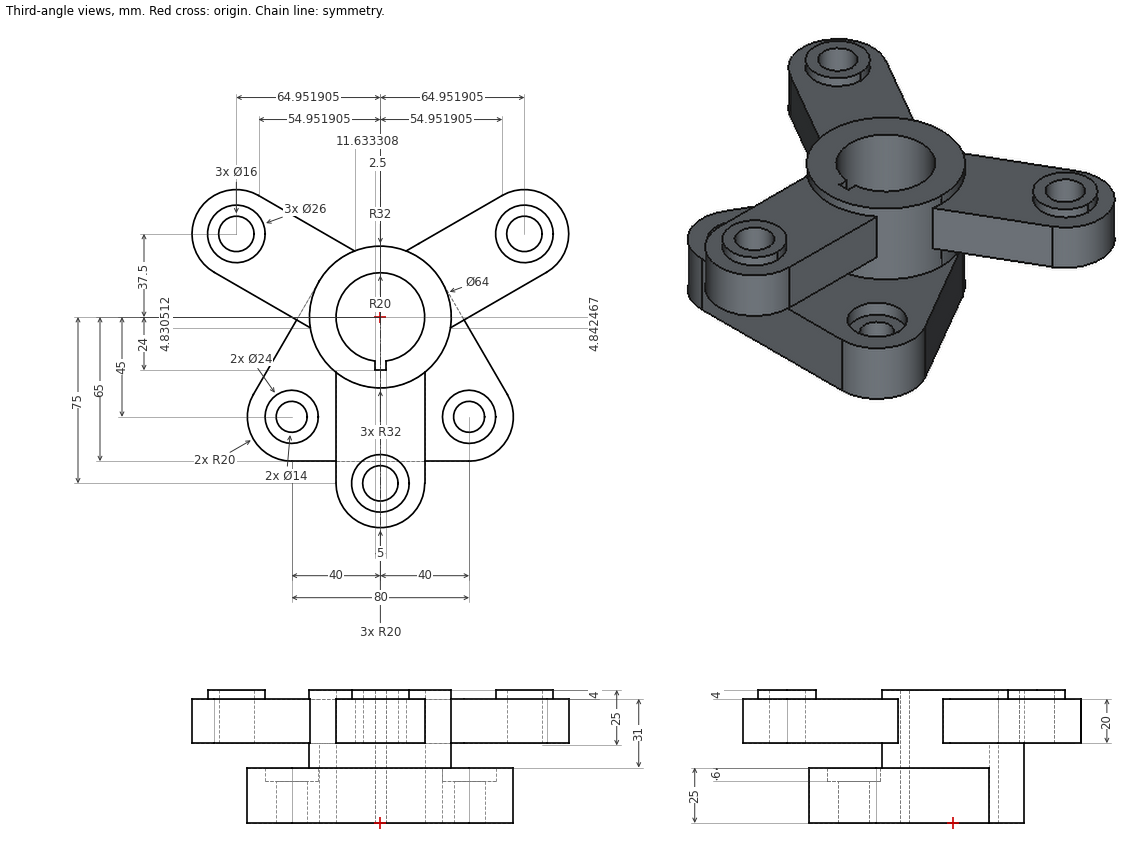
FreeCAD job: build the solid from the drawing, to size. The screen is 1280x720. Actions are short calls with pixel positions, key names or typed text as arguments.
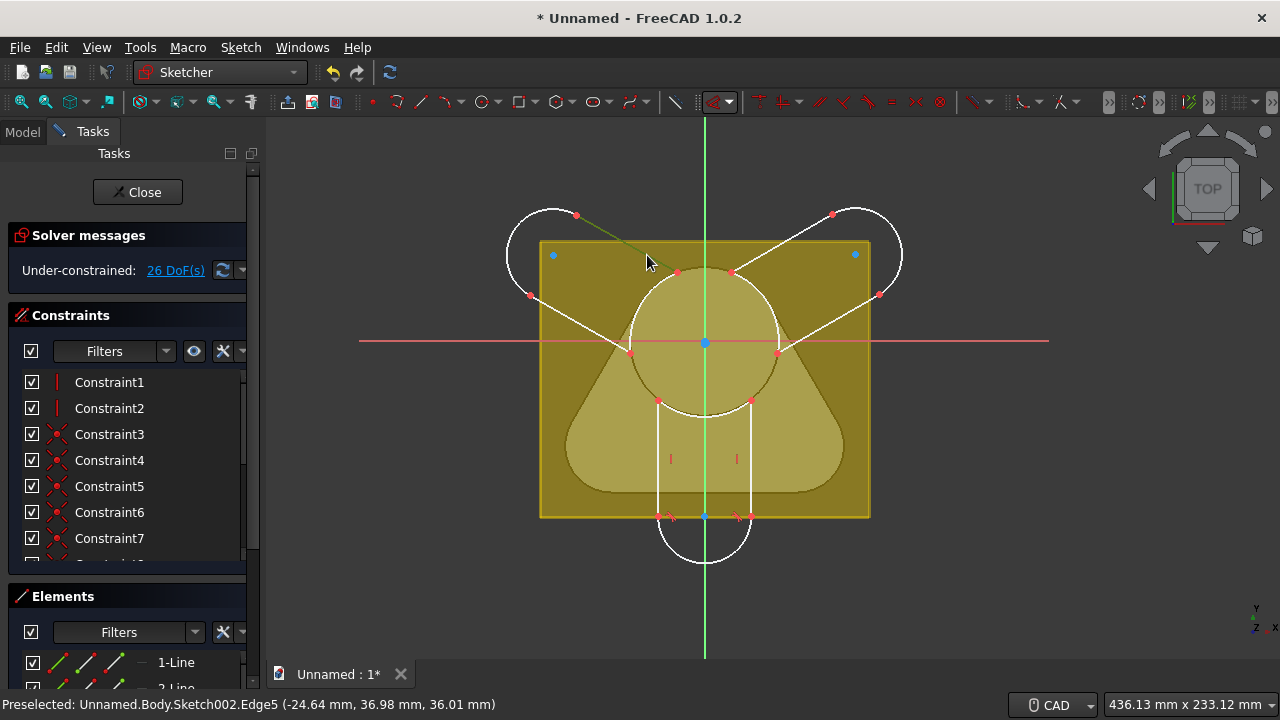
click(534, 213)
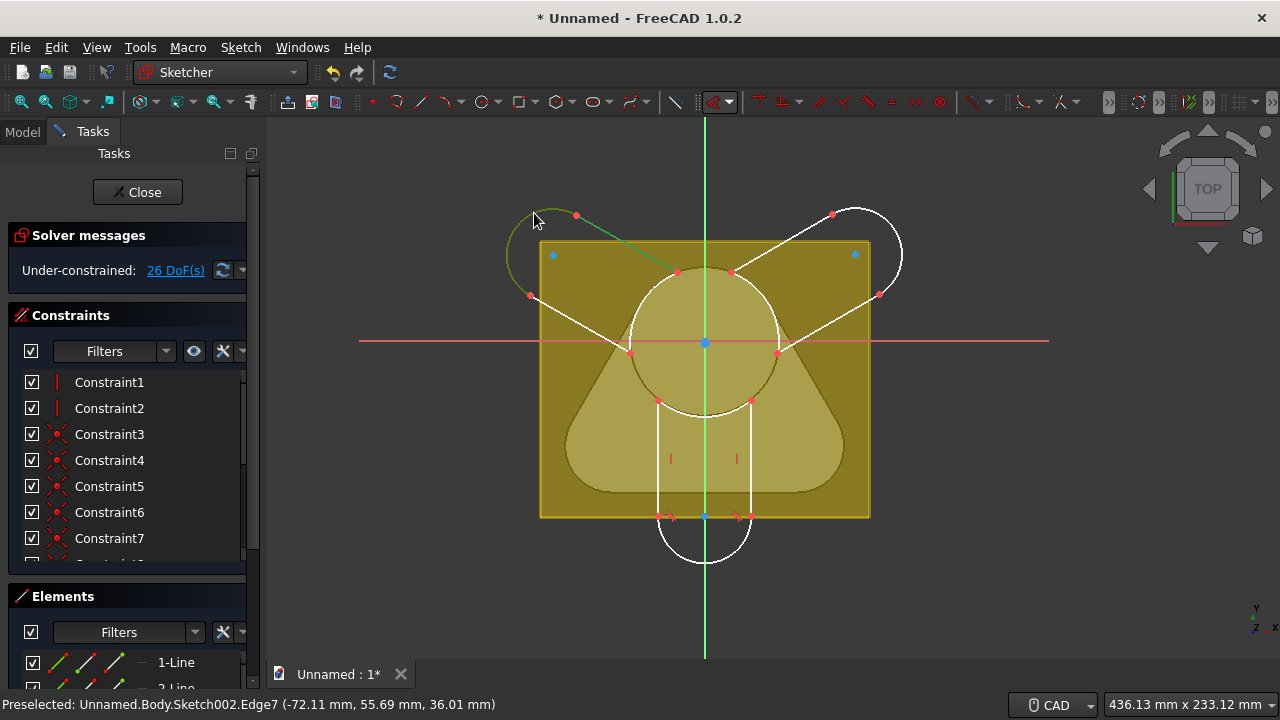
key(t)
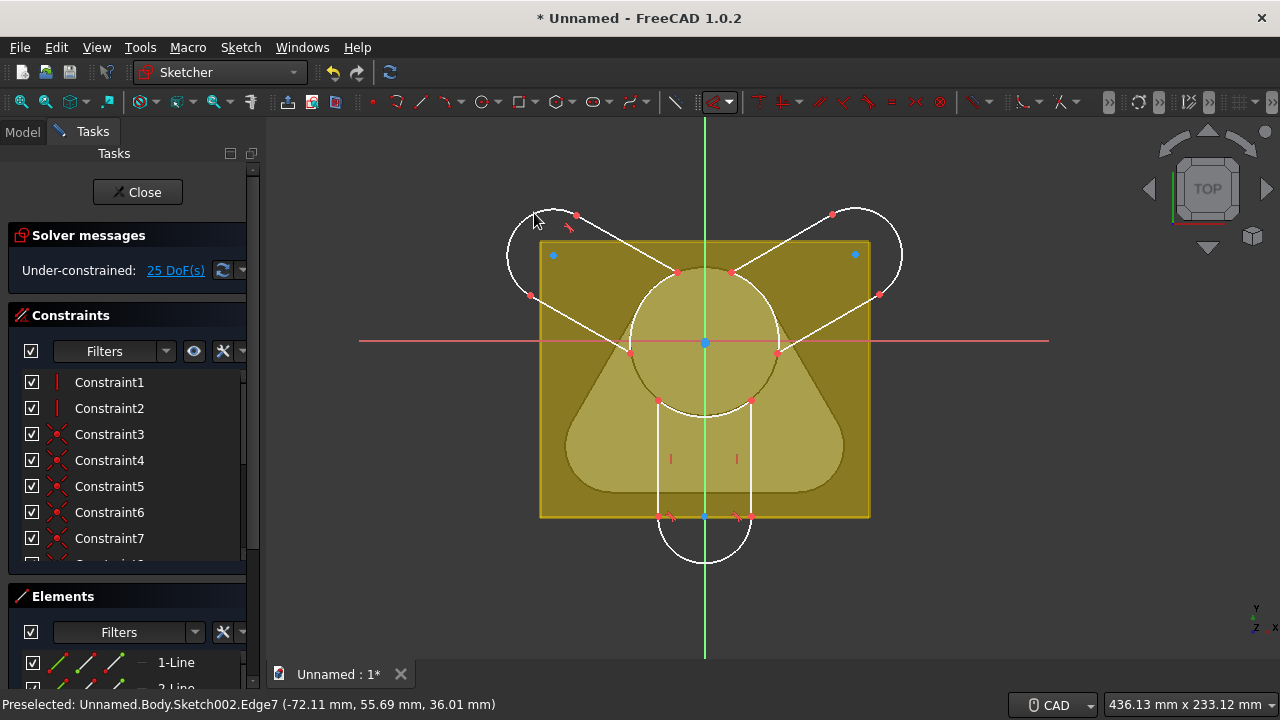
click(560, 313)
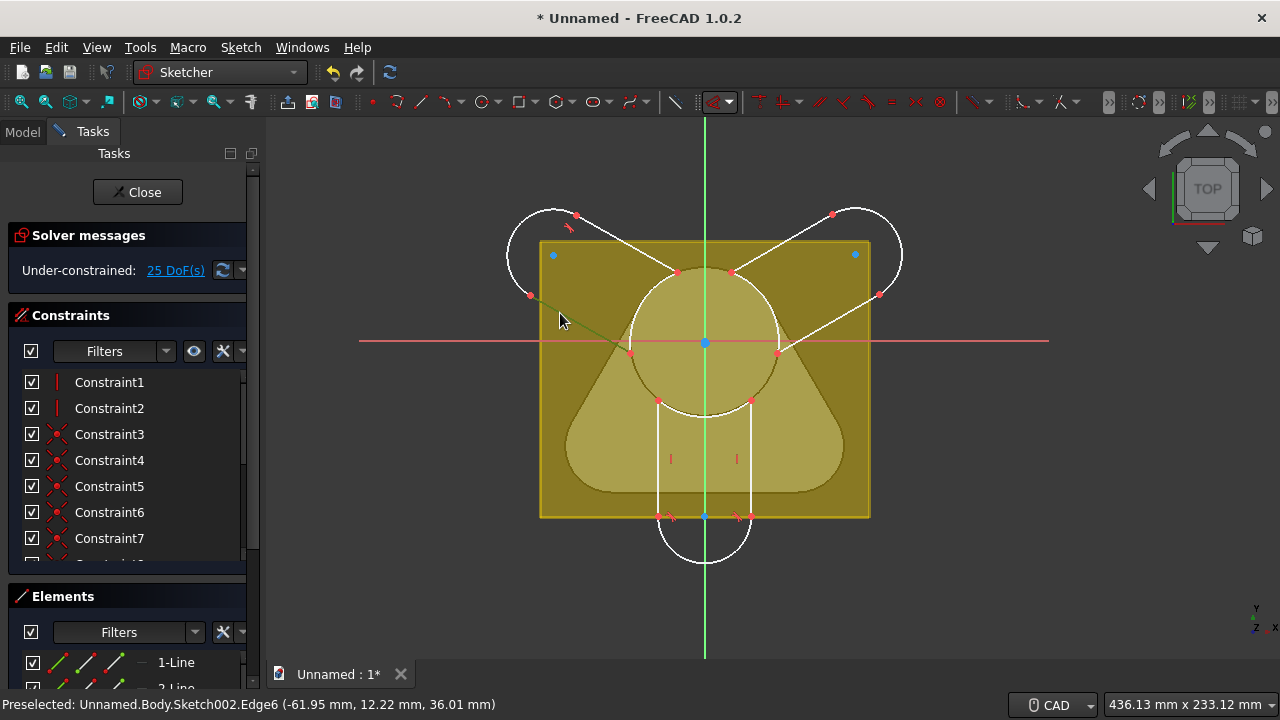
click(535, 214)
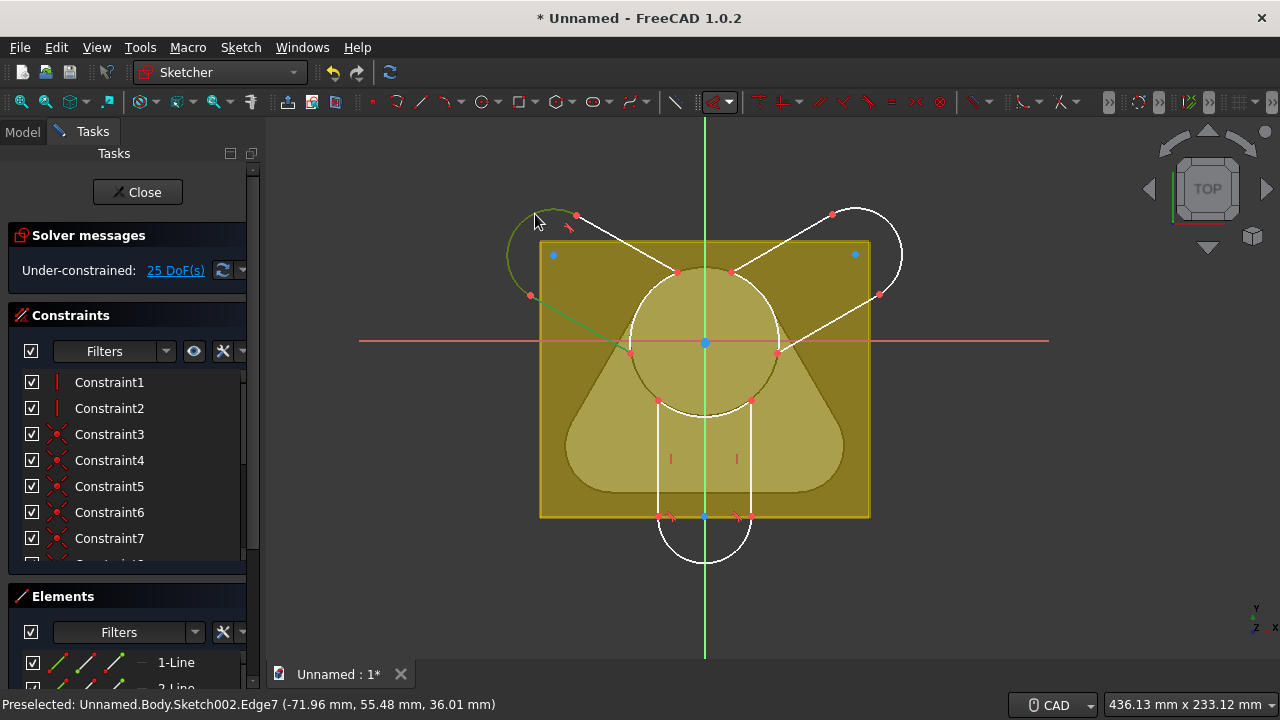
key(t)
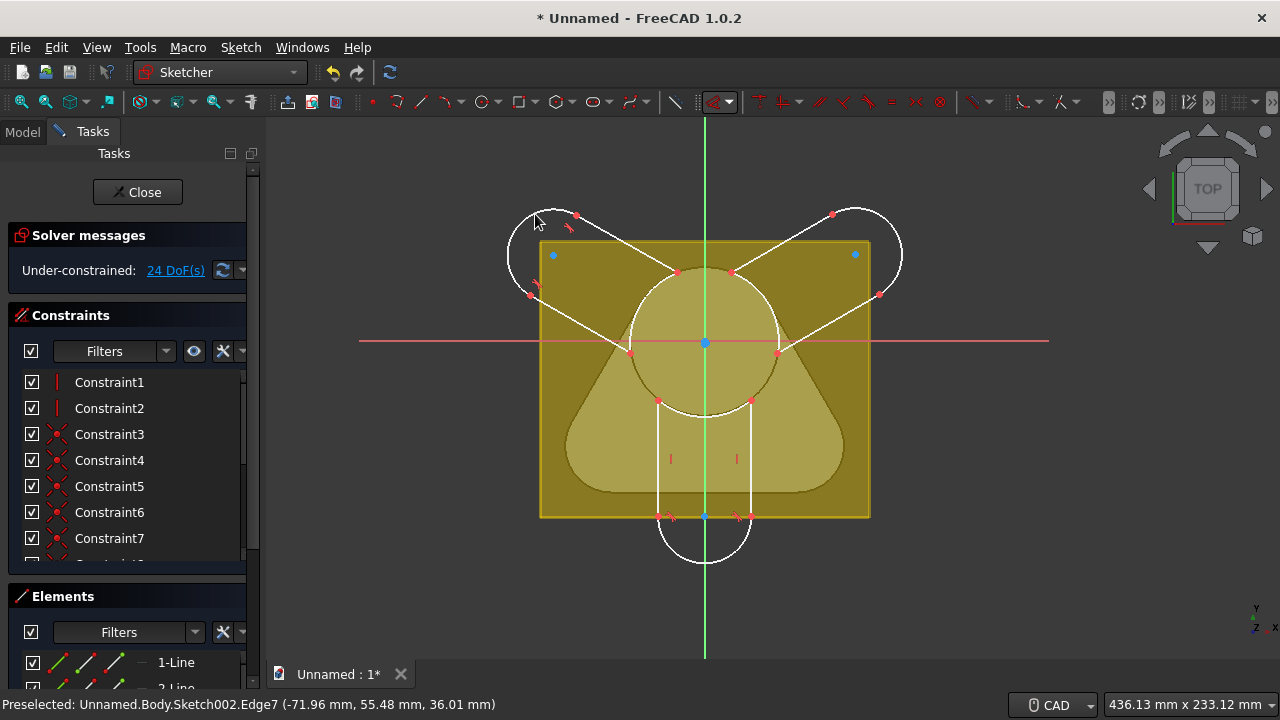
click(802, 232)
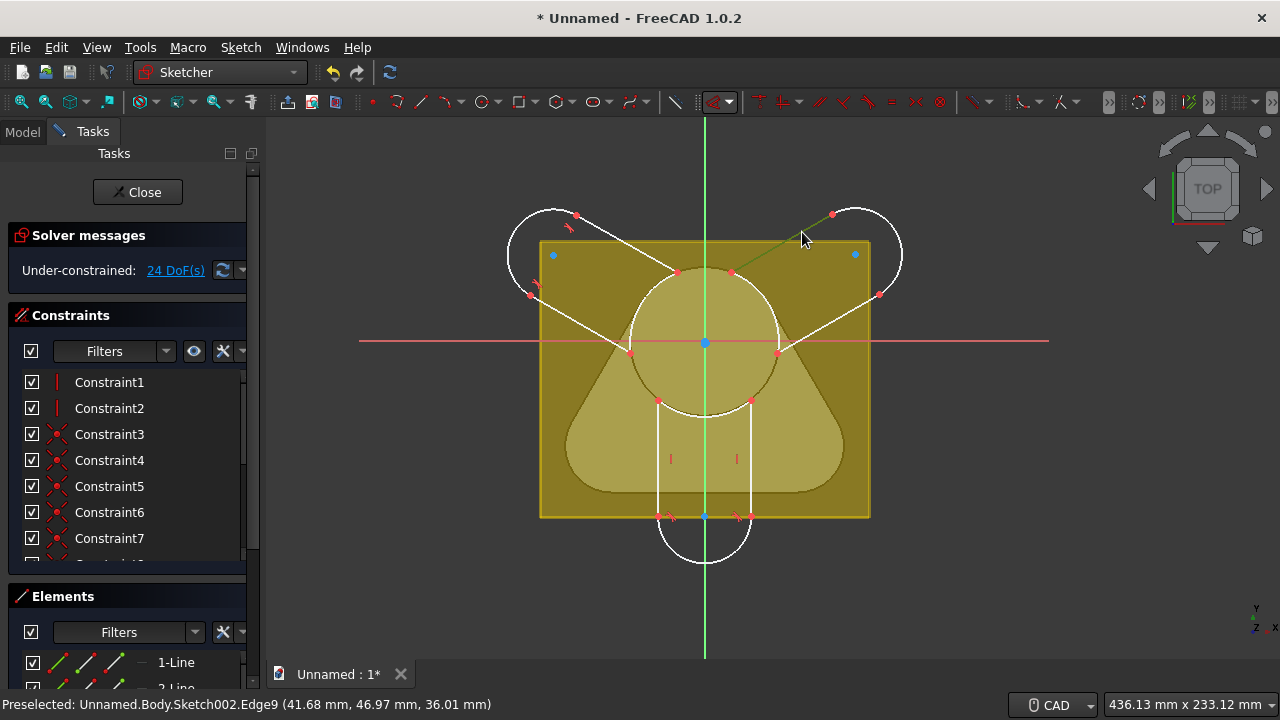
click(902, 259)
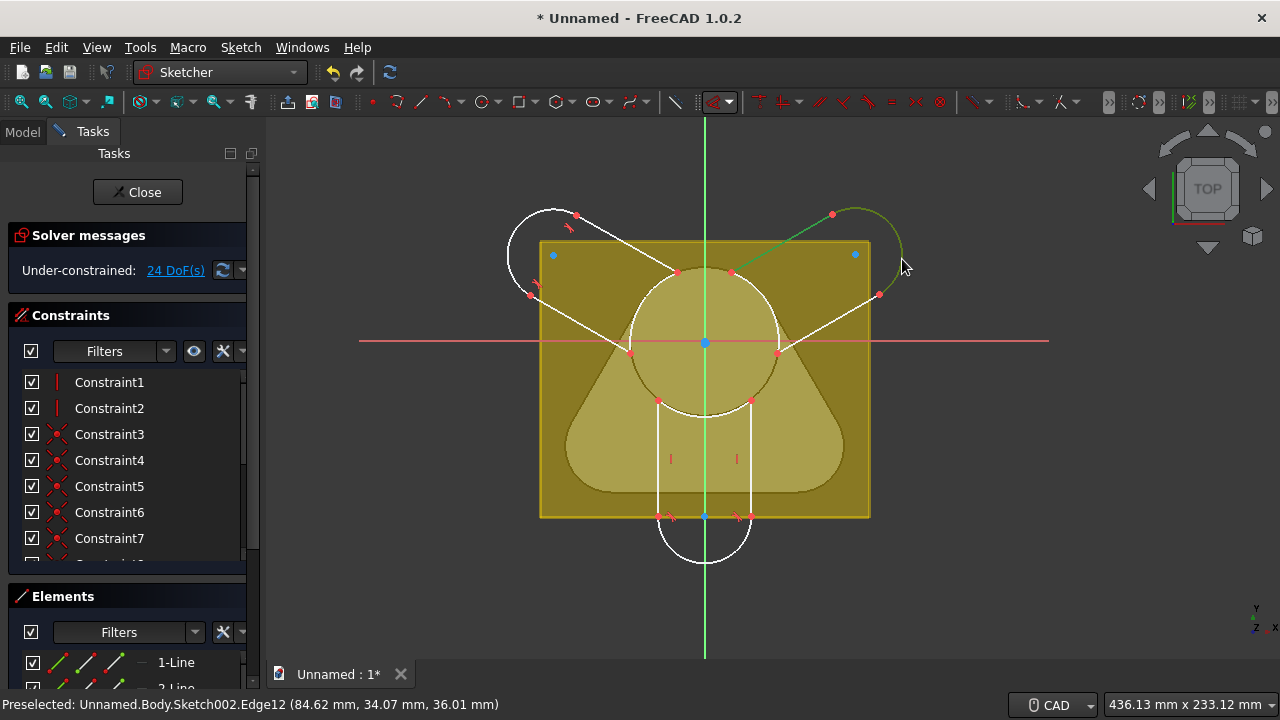
key(t)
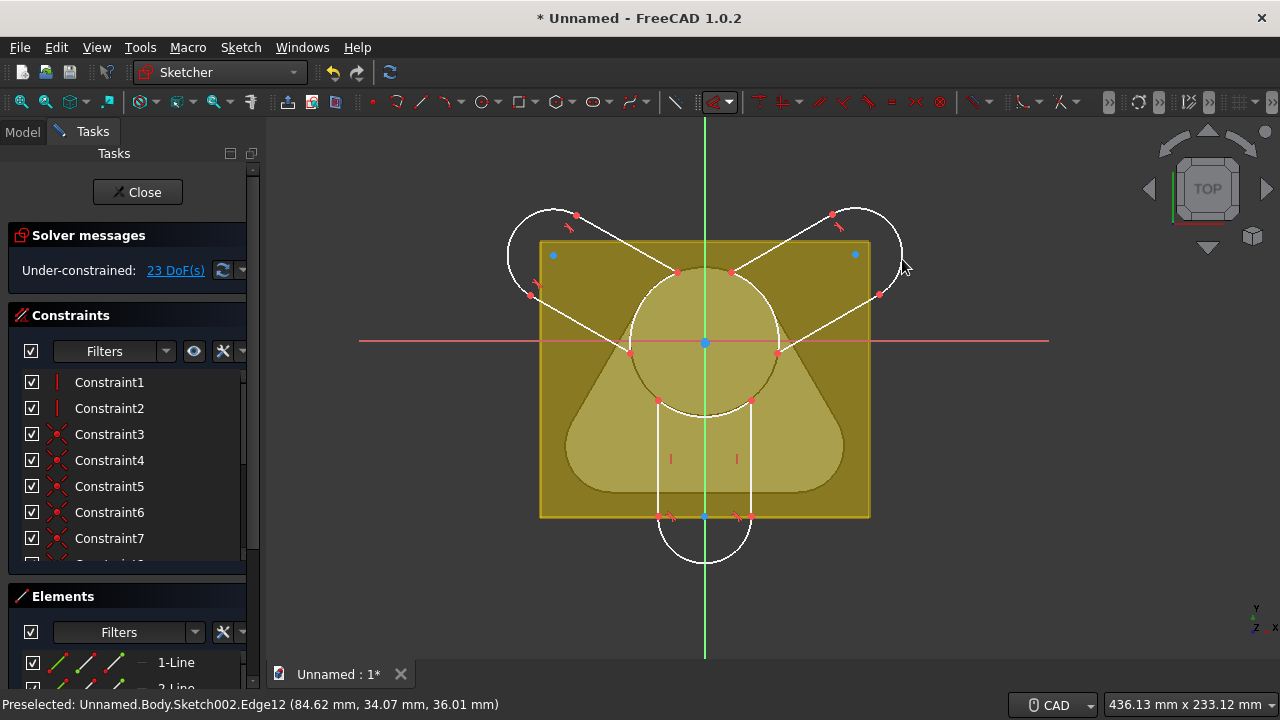
click(849, 312)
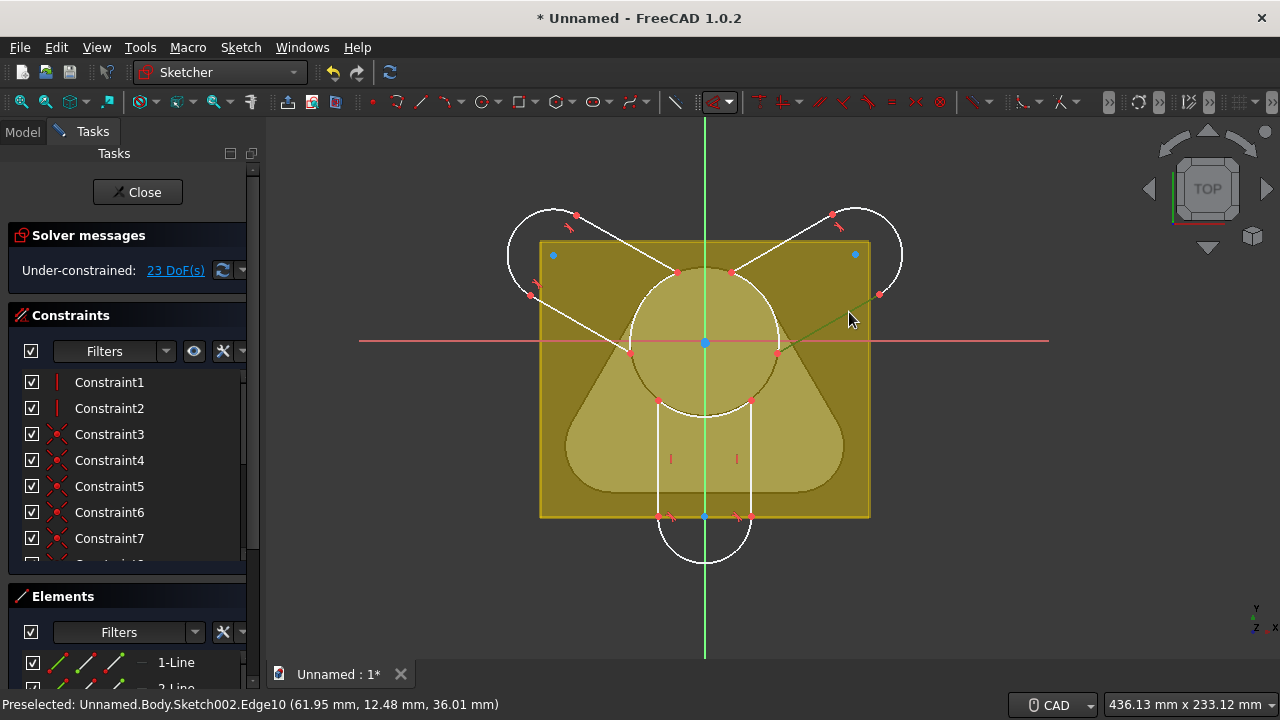
click(902, 259)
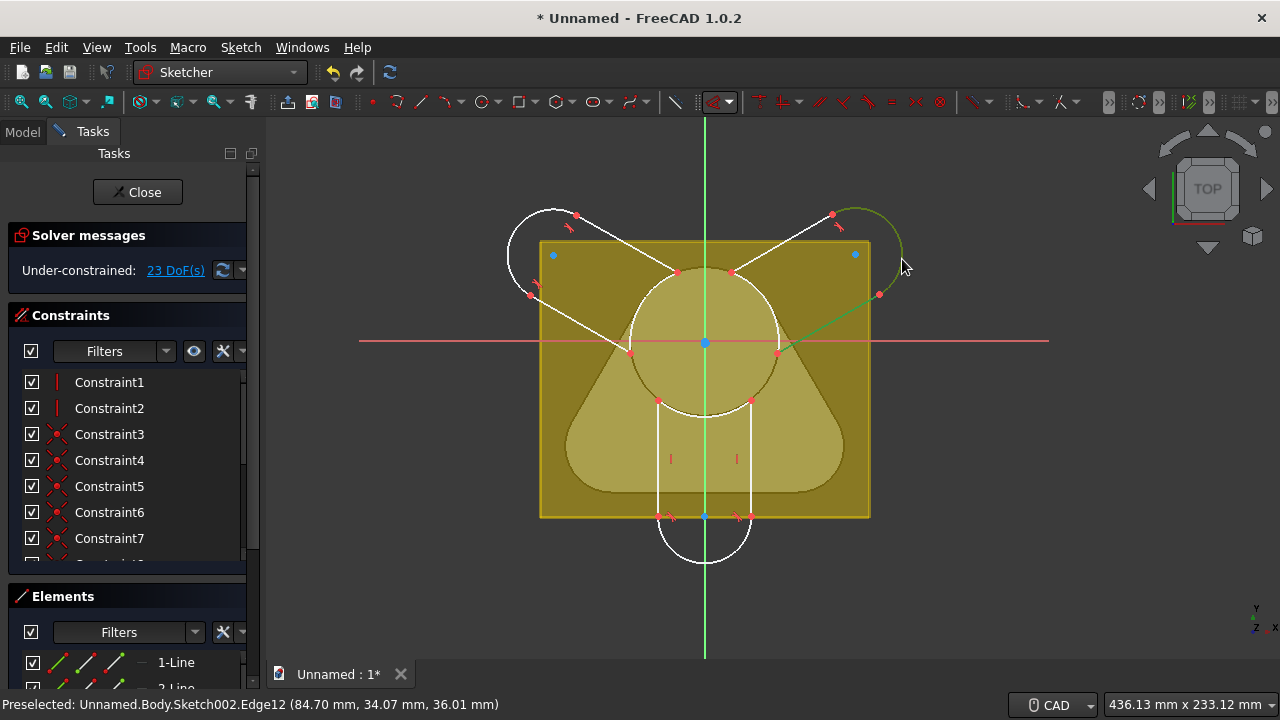
key(t)